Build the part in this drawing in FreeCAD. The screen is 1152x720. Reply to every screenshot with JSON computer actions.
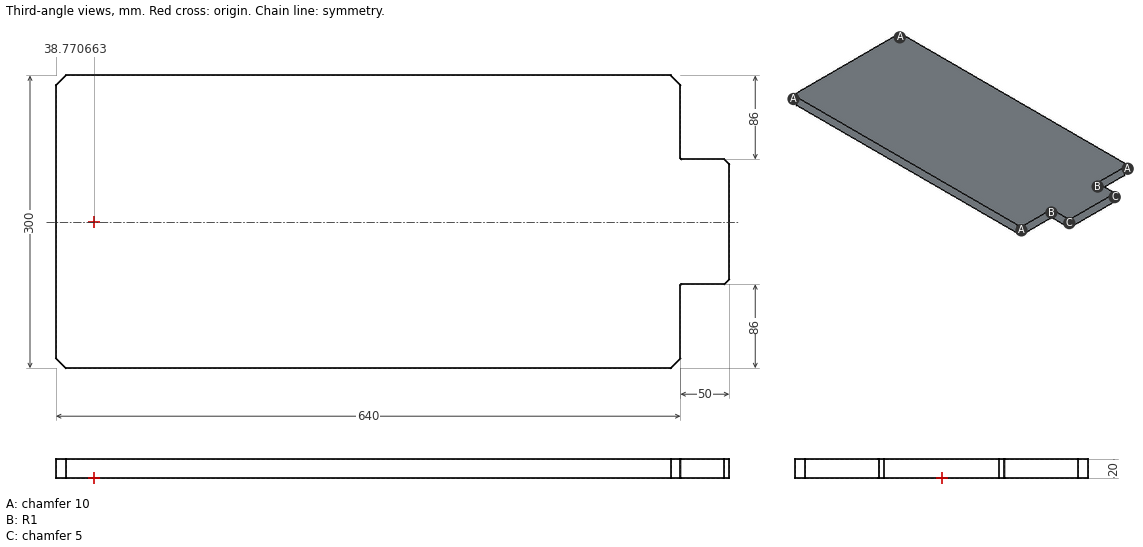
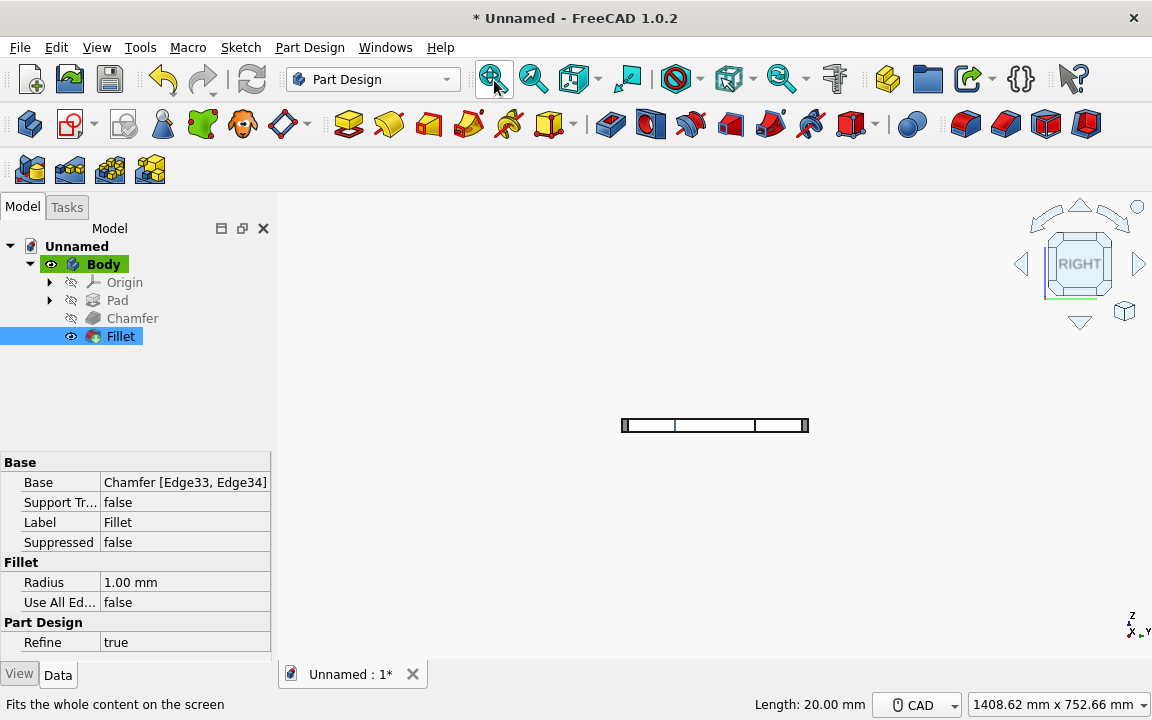
{"action": "left_click", "coordinate": [494, 80]}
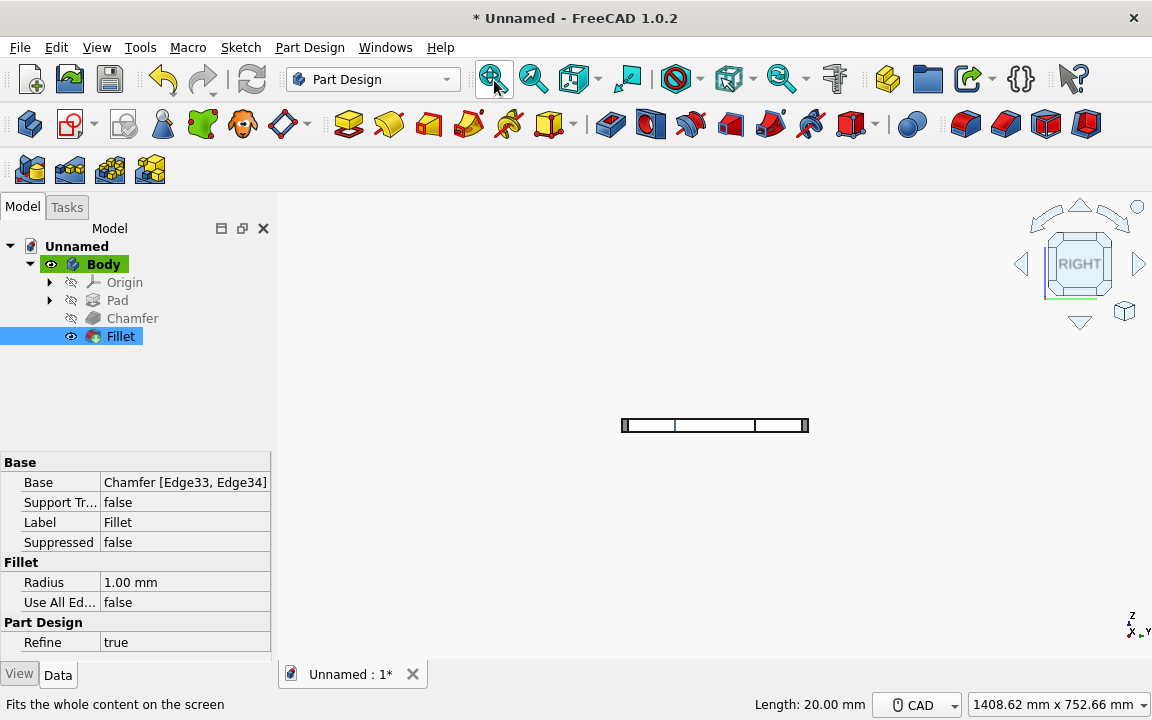
{"action": "scroll", "coordinate": [755, 424], "scroll_direction": "up", "scroll_amount": 6}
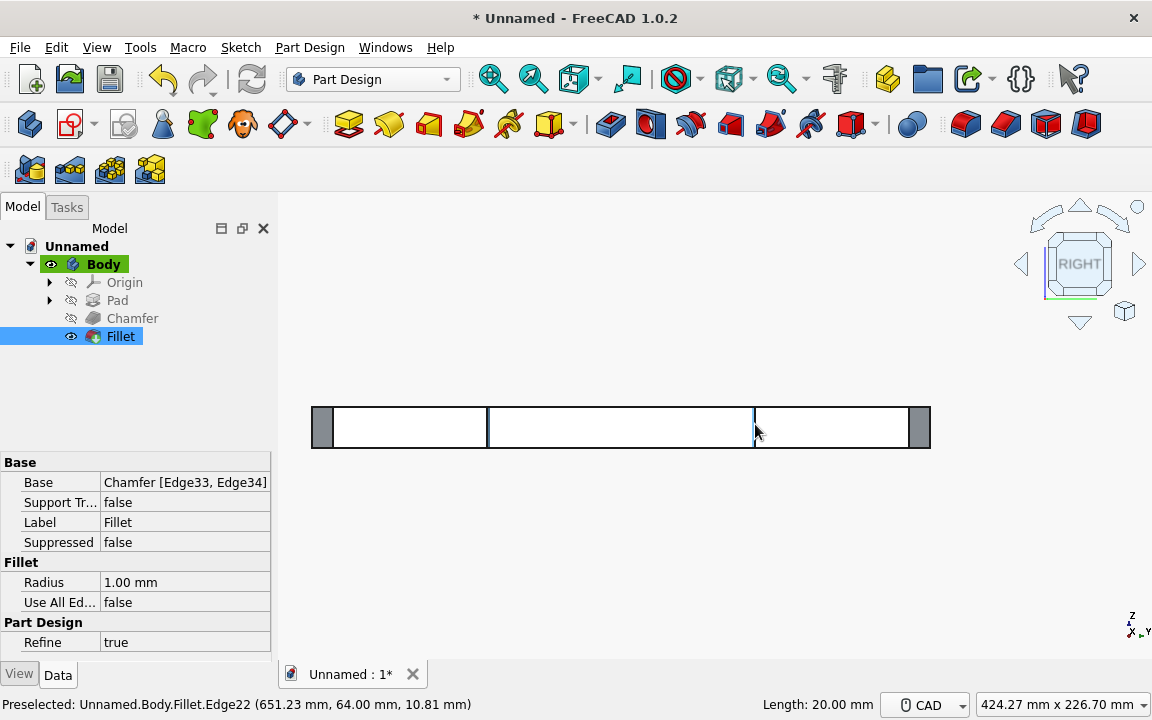
{"action": "left_click", "coordinate": [753, 427], "text": "ctrl"}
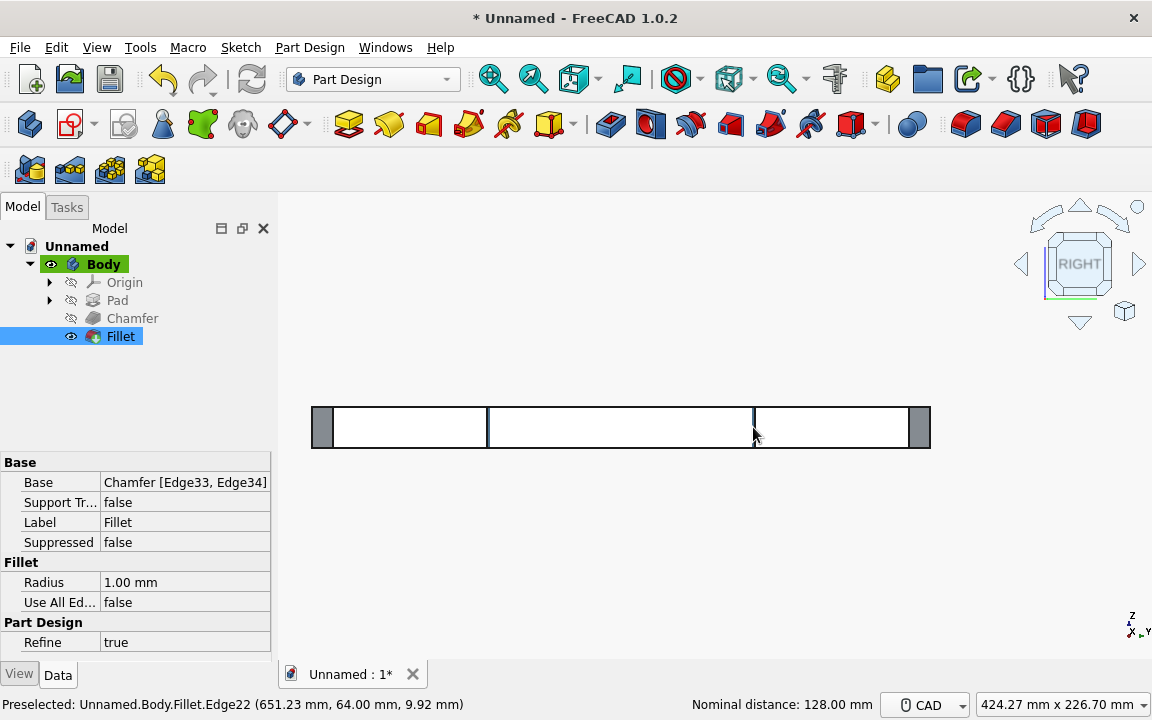
{"action": "left_click", "coordinate": [1006, 124]}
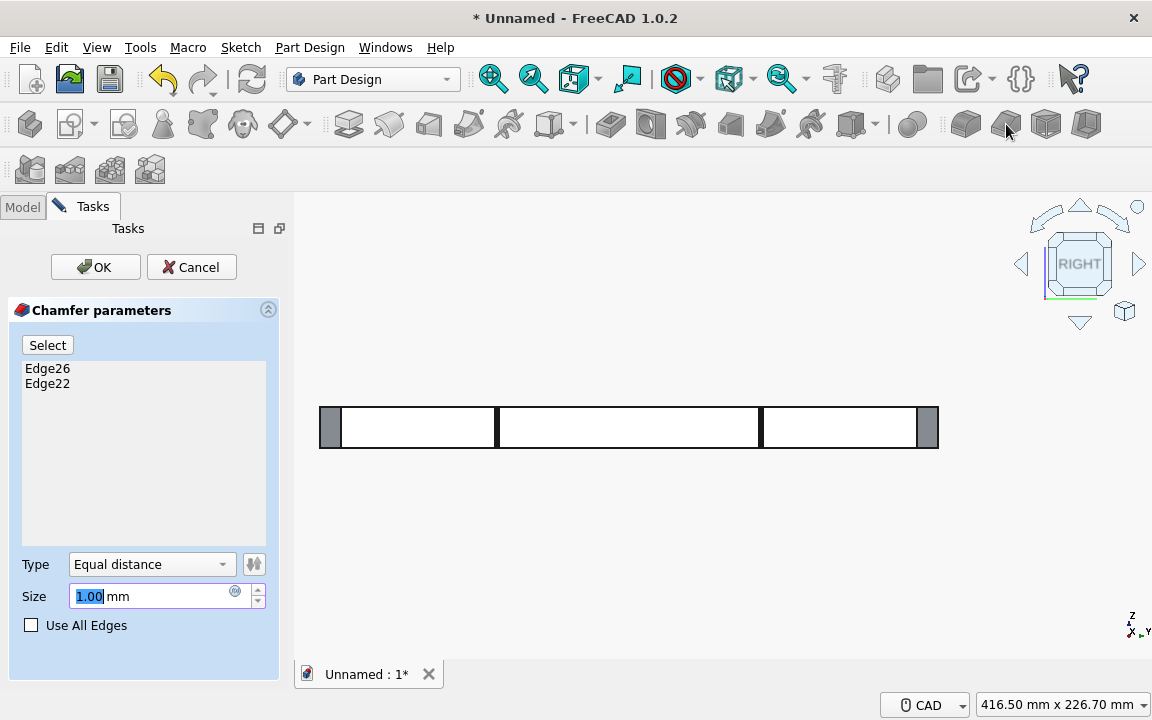
{"action": "type", "text": "5"}
{"action": "key", "text": "Tab"}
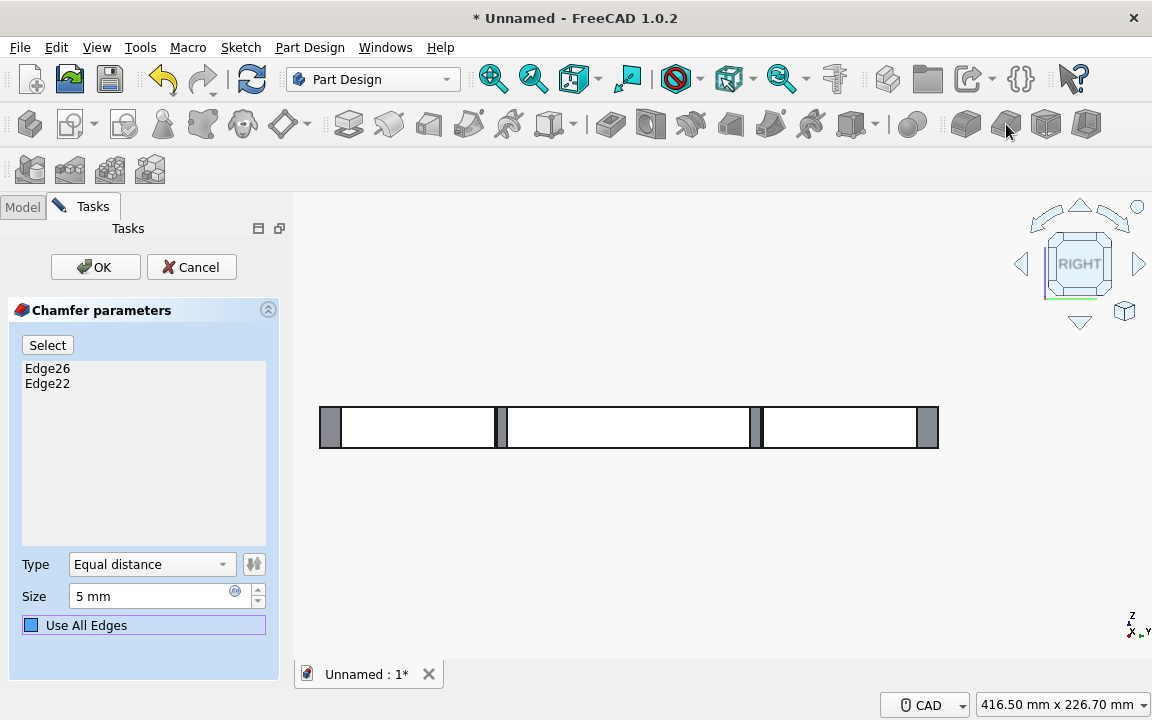
{"action": "left_click", "coordinate": [96, 267]}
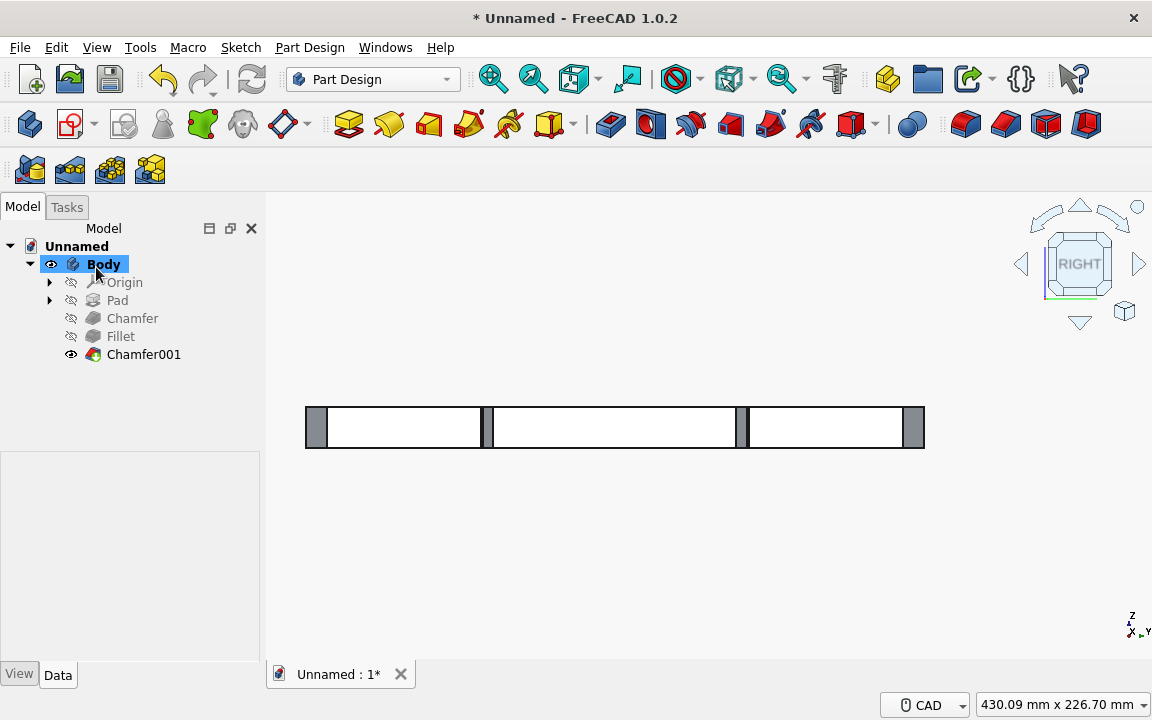
{"action": "key", "text": "0"}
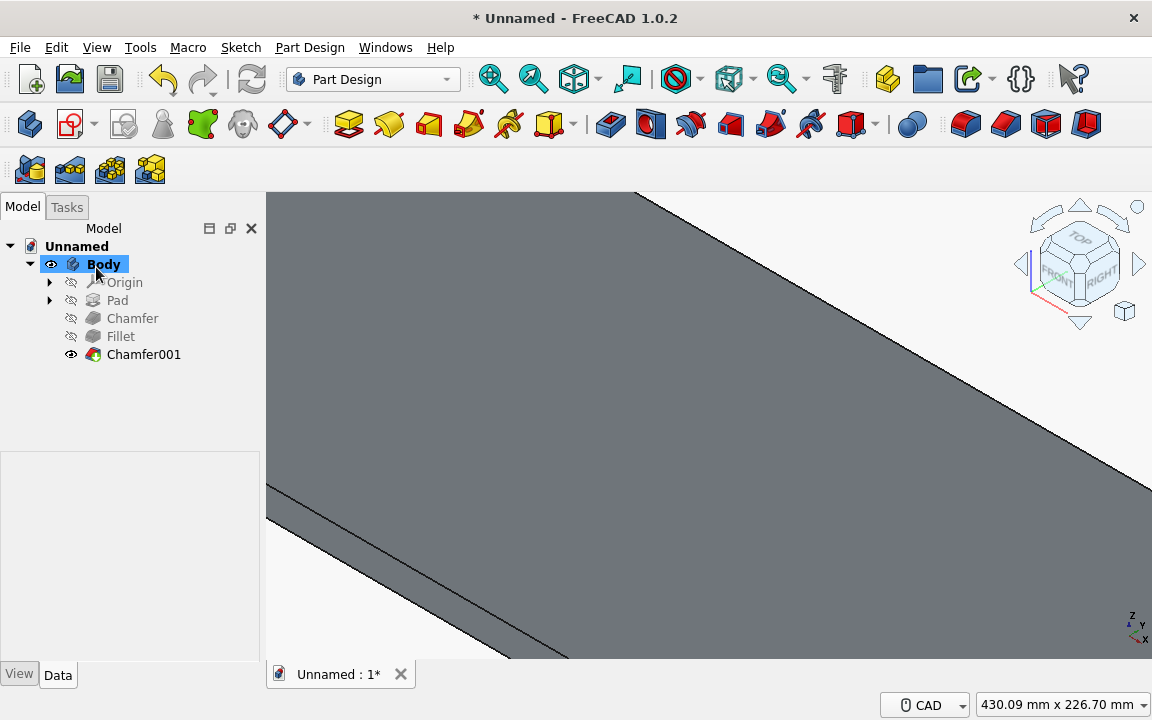
{"action": "left_click", "coordinate": [494, 80]}